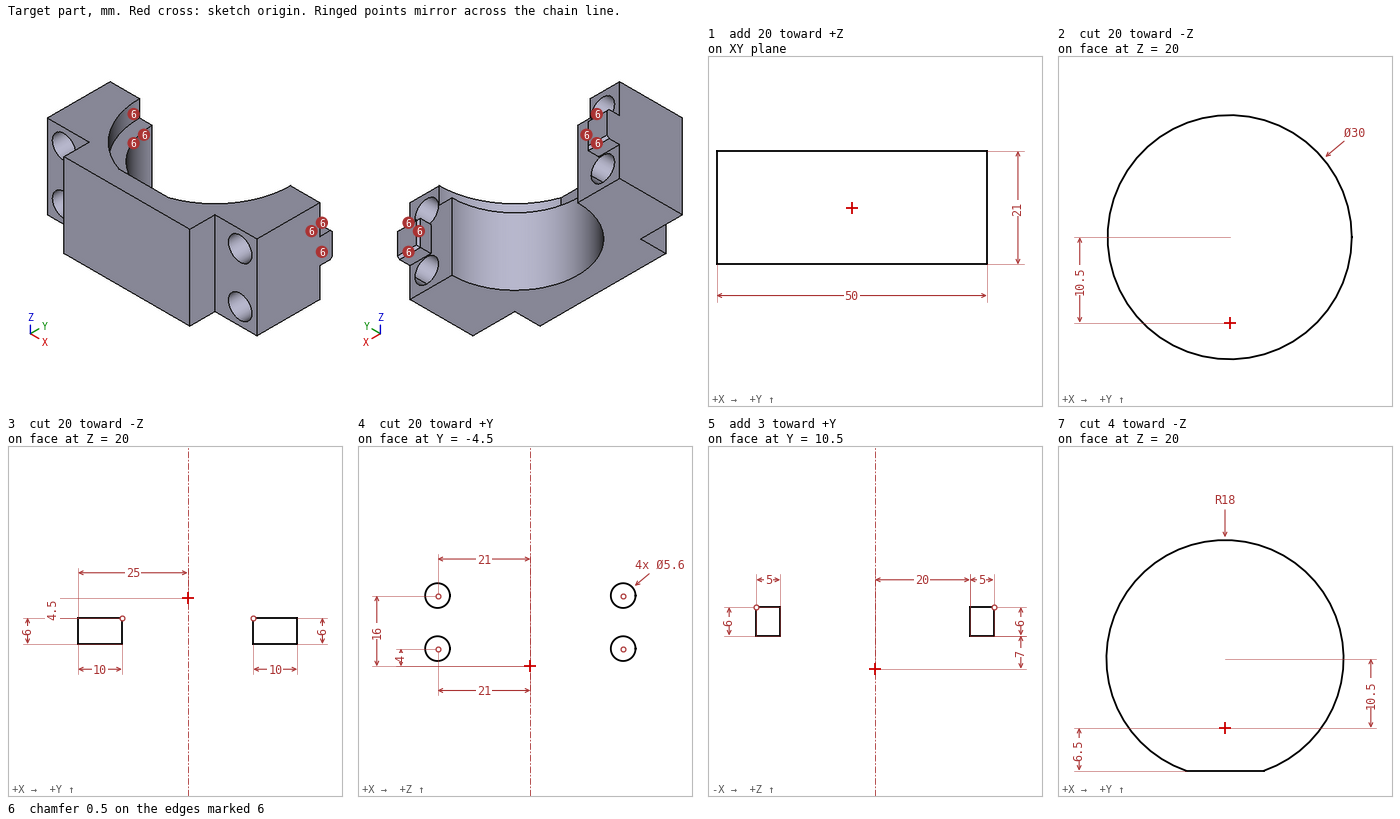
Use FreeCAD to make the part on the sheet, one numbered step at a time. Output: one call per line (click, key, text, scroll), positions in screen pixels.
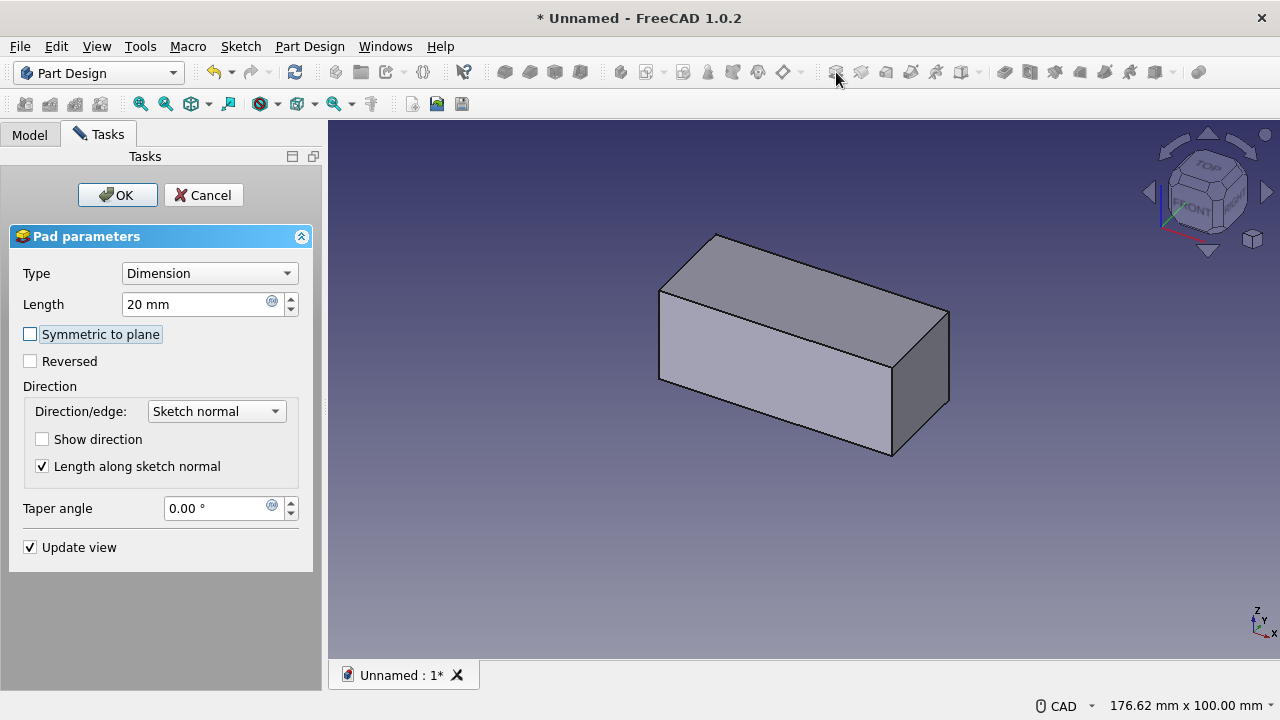
click(118, 195)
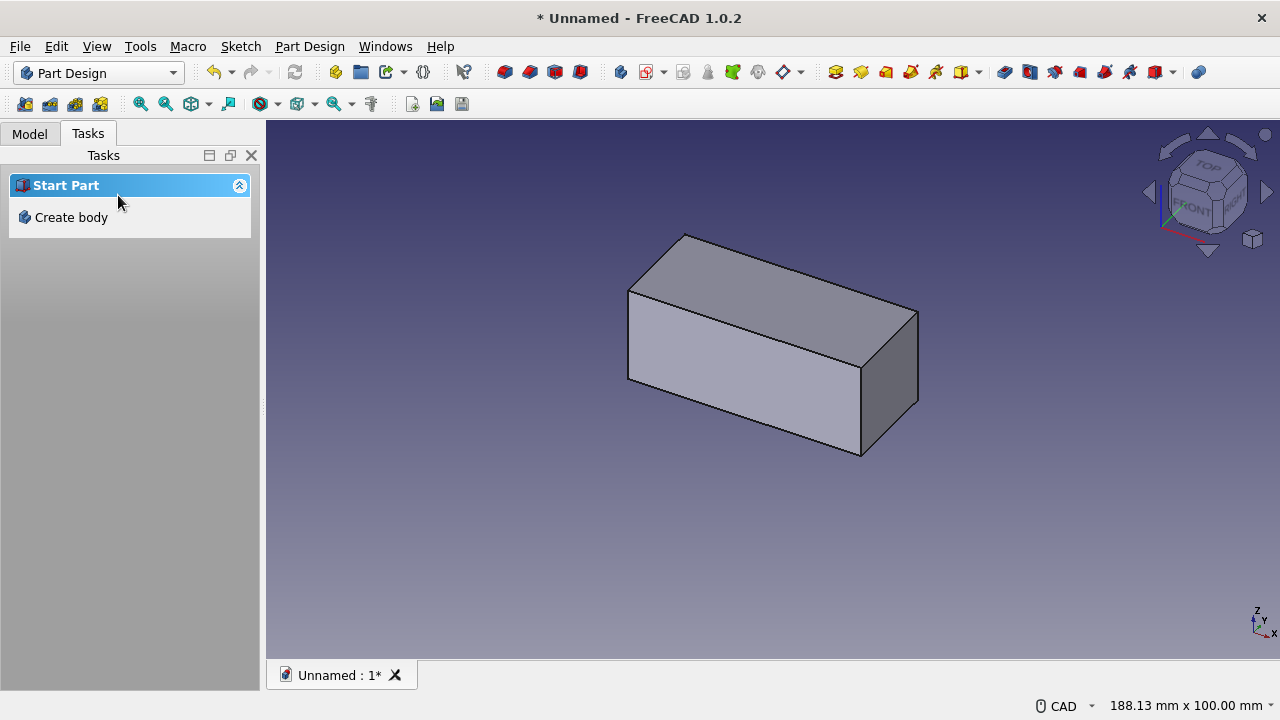
key(v)
key(f)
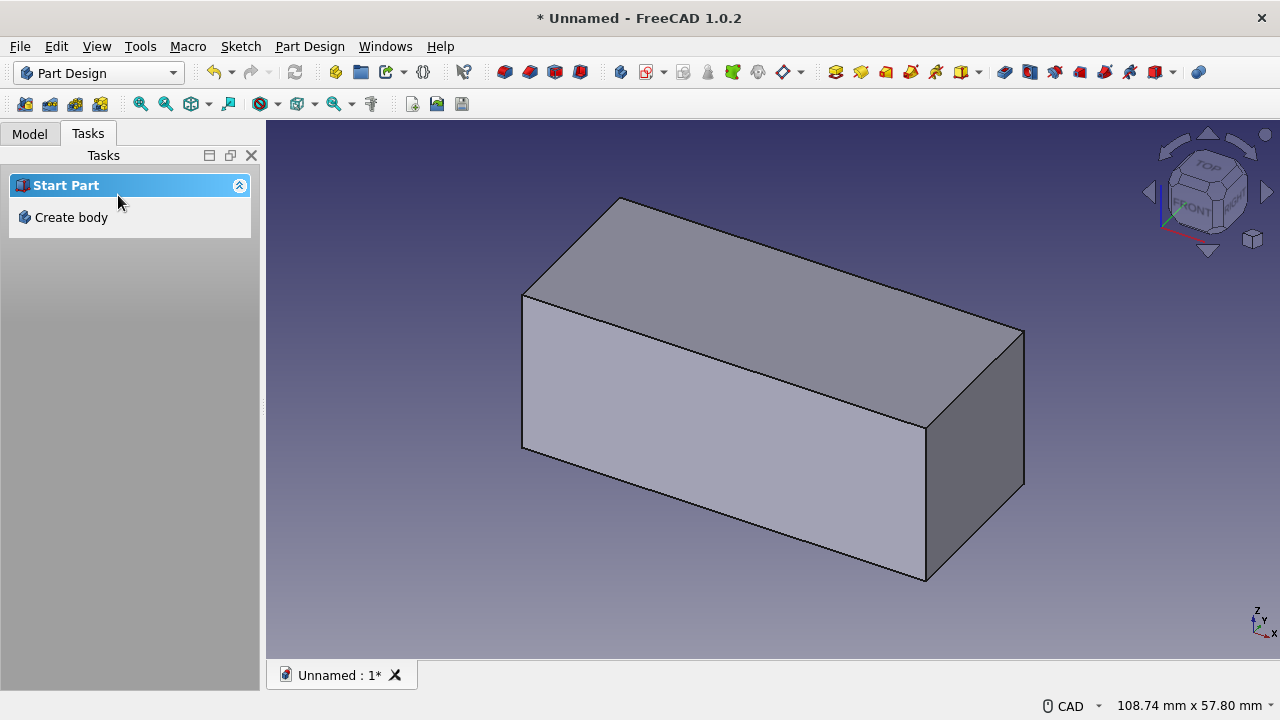
click(888, 350)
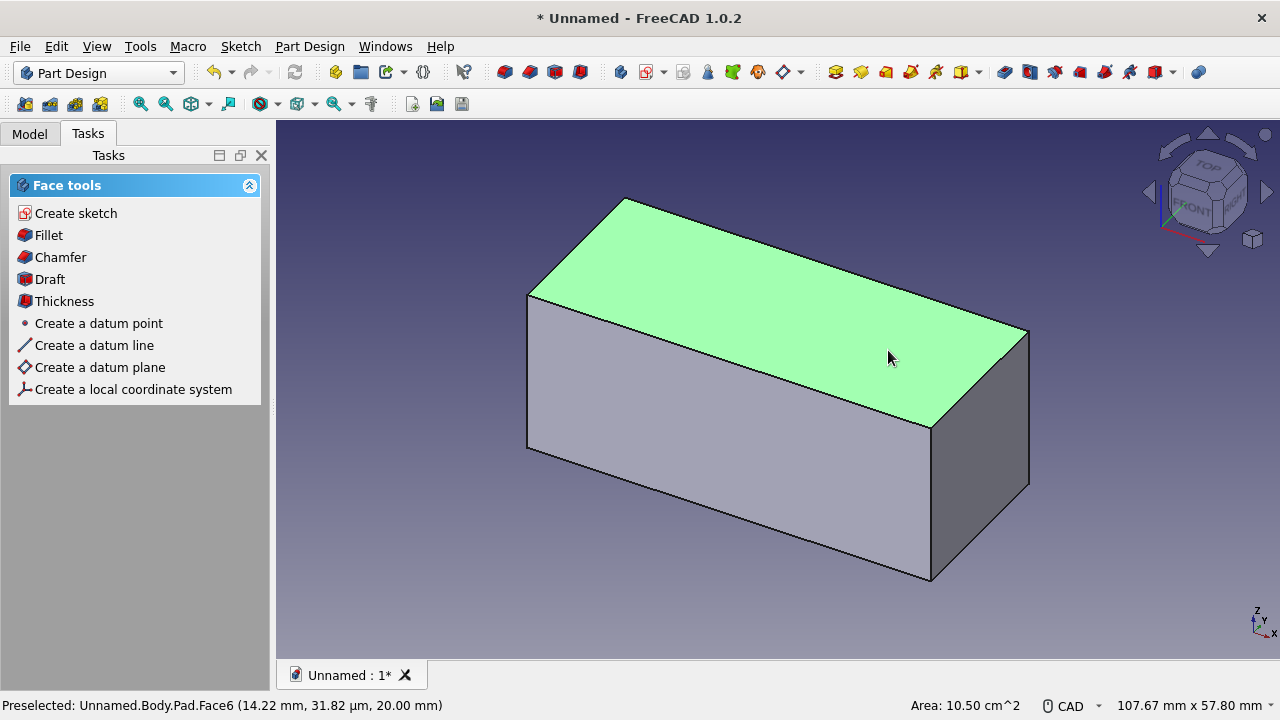
click(646, 72)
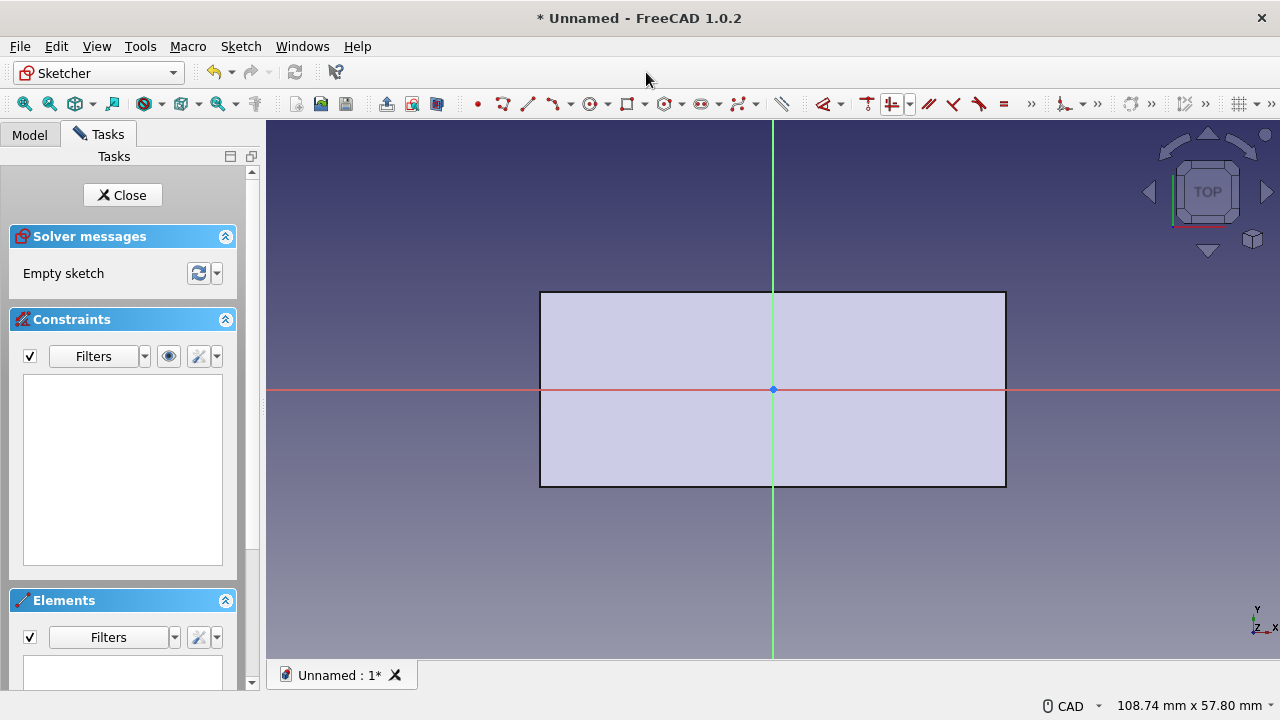
scroll(395, 631, down, 1)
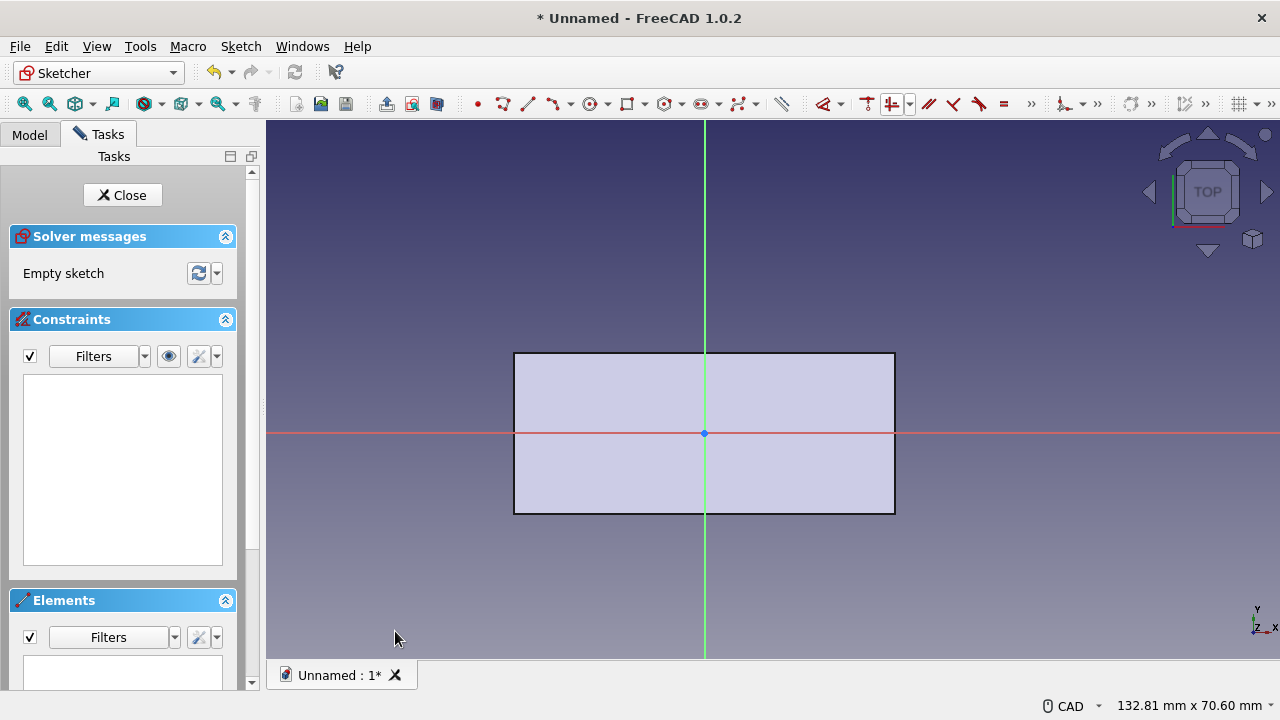
scroll(705, 280, up, 2)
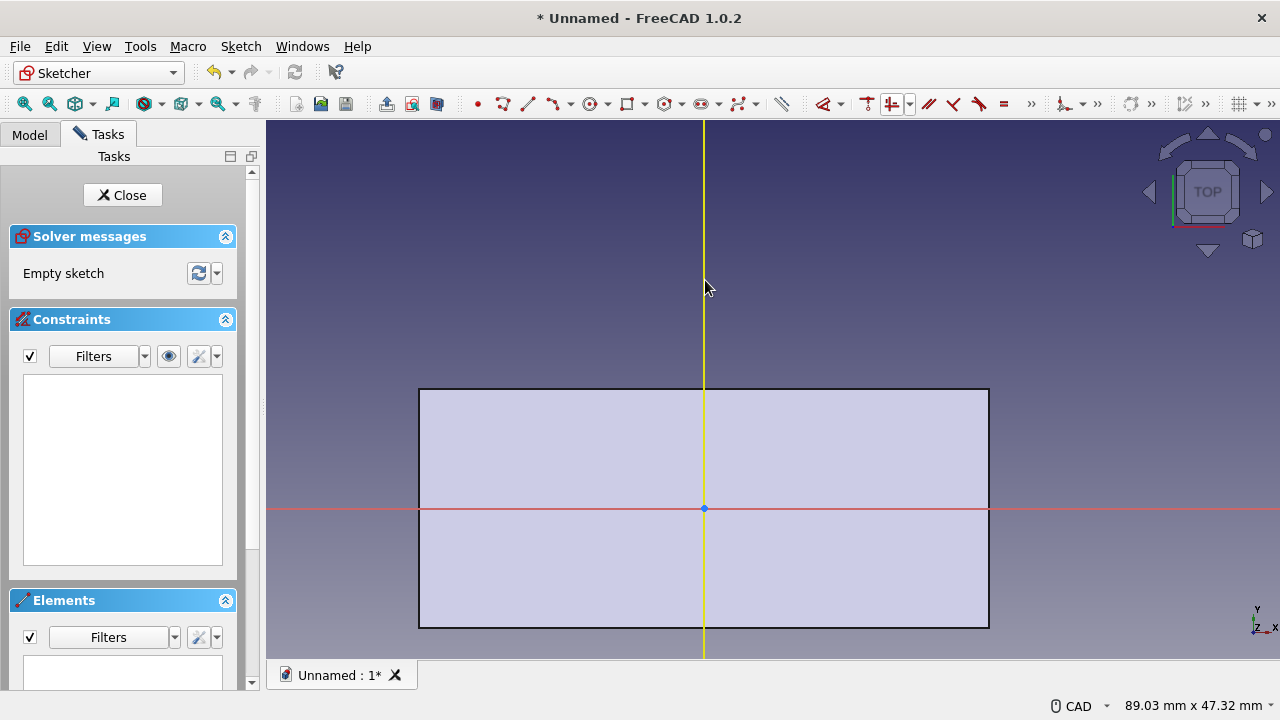
key(g)
key(c)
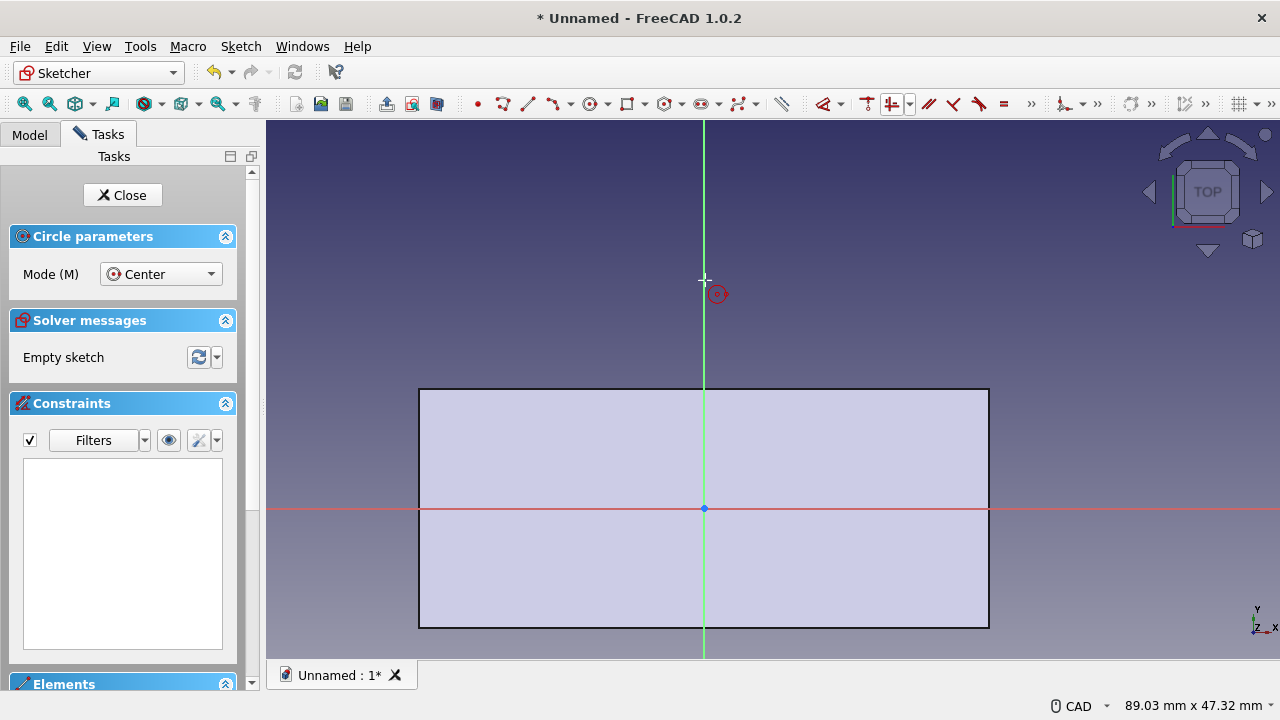
click(704, 389)
move(825, 268)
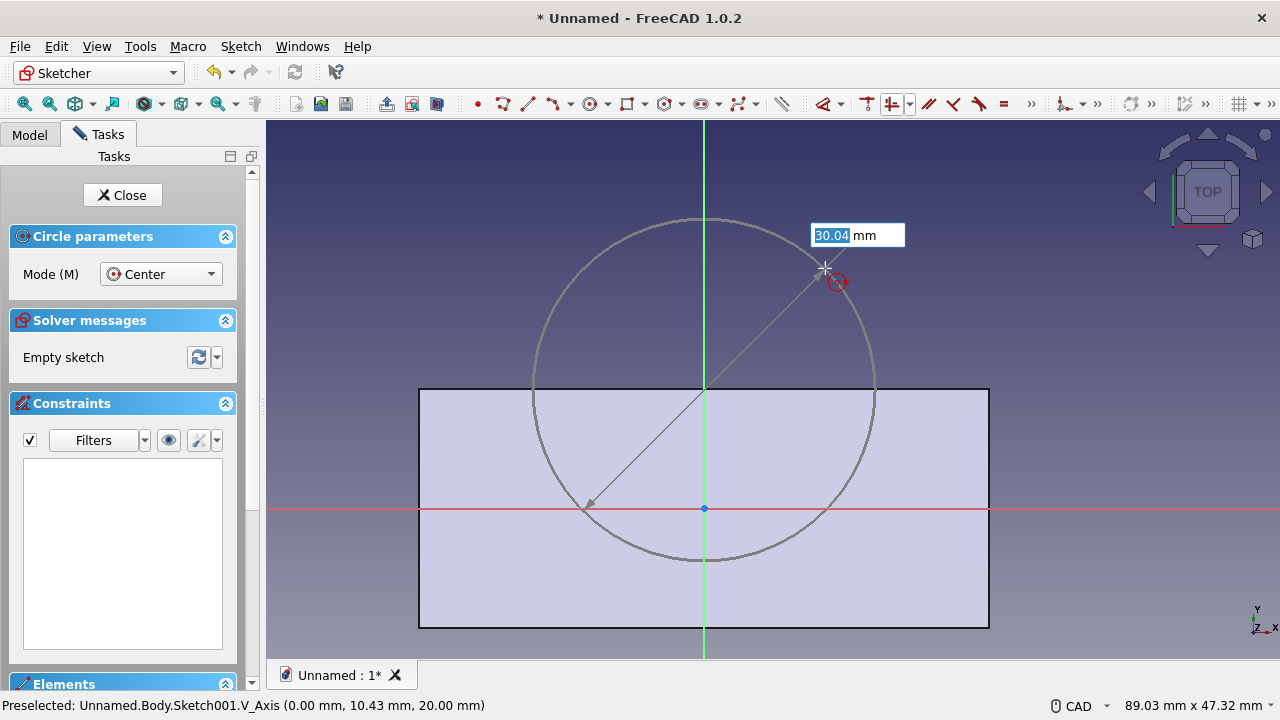
text(30)
key(Return)
key(Escape)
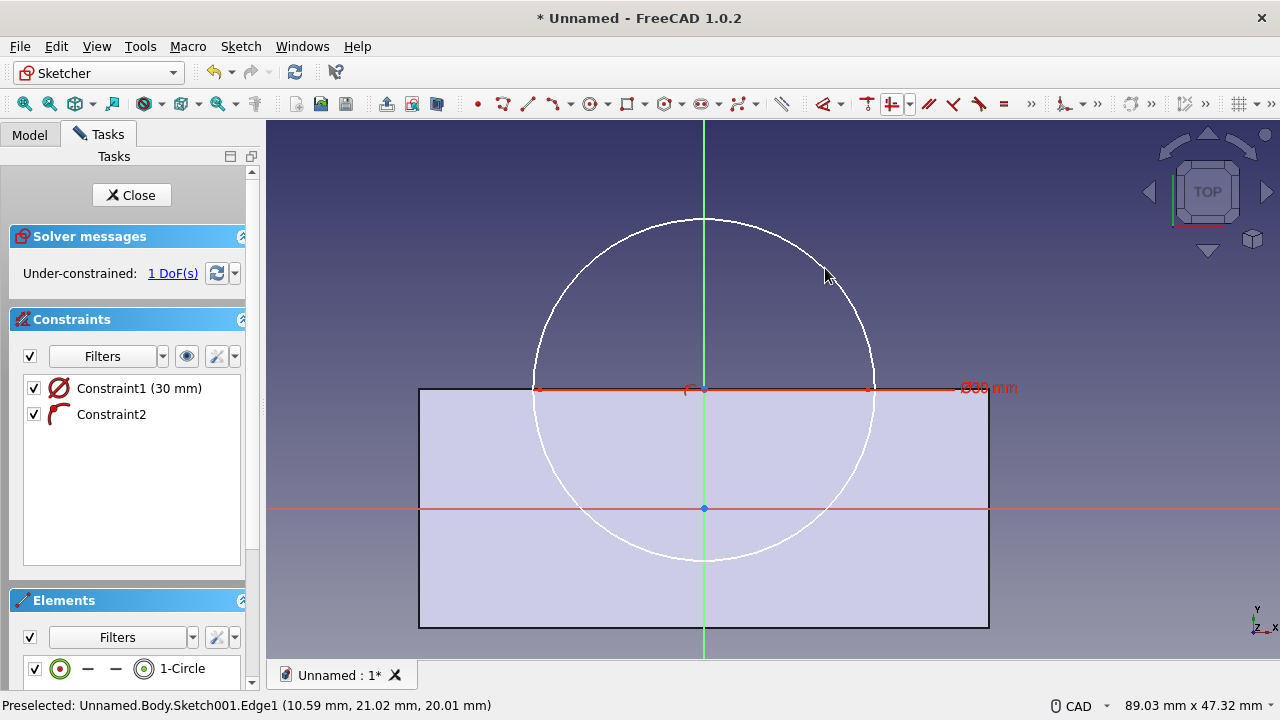
click(822, 104)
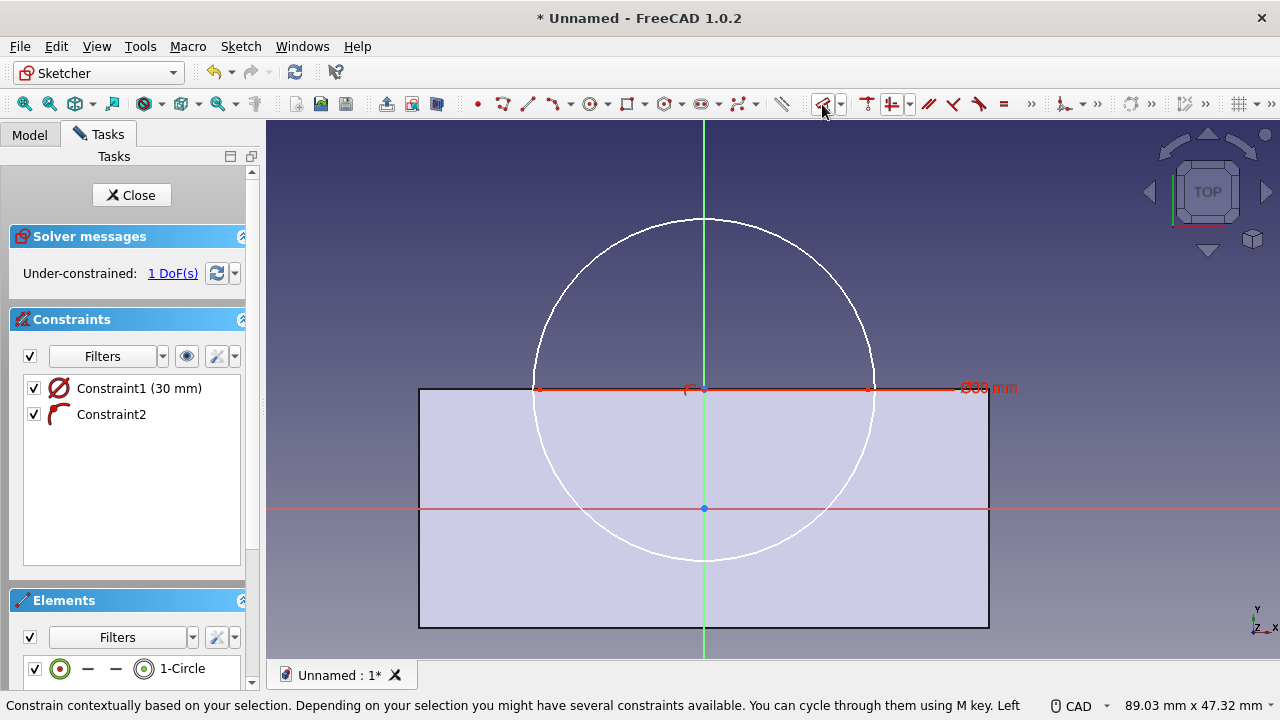
click(704, 390)
click(738, 449)